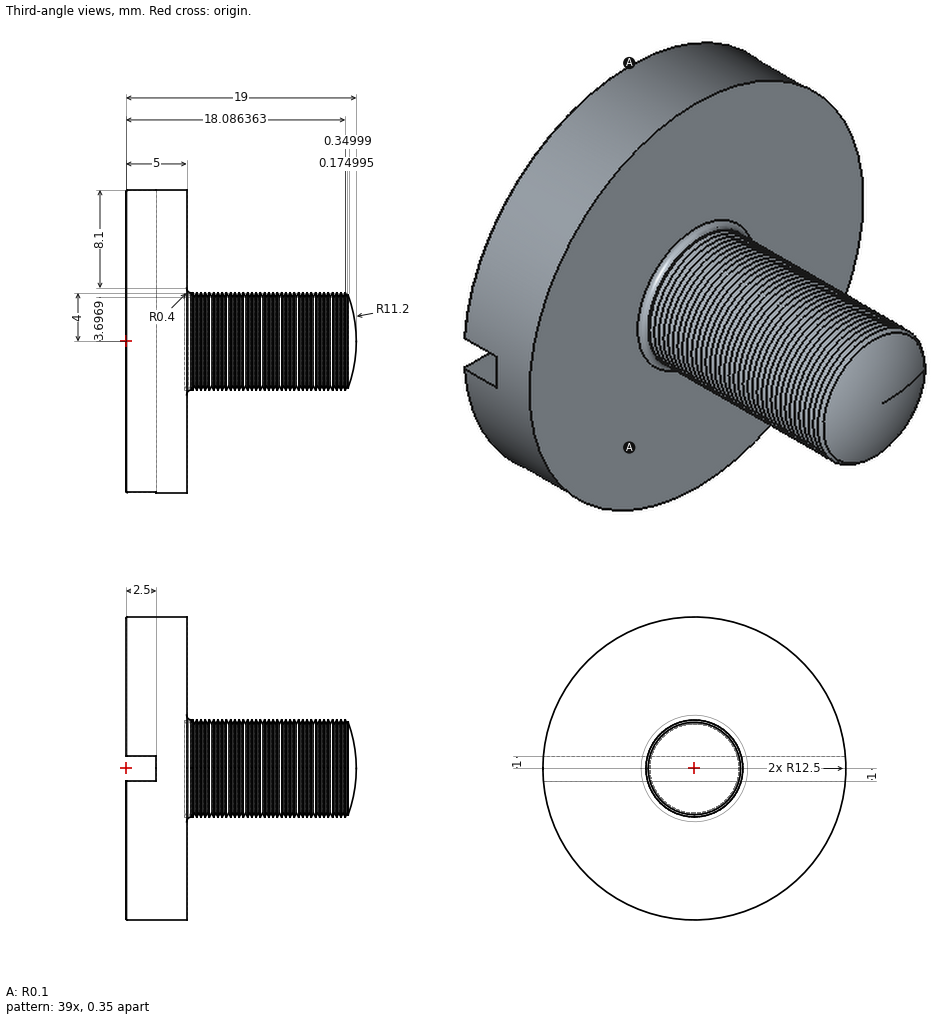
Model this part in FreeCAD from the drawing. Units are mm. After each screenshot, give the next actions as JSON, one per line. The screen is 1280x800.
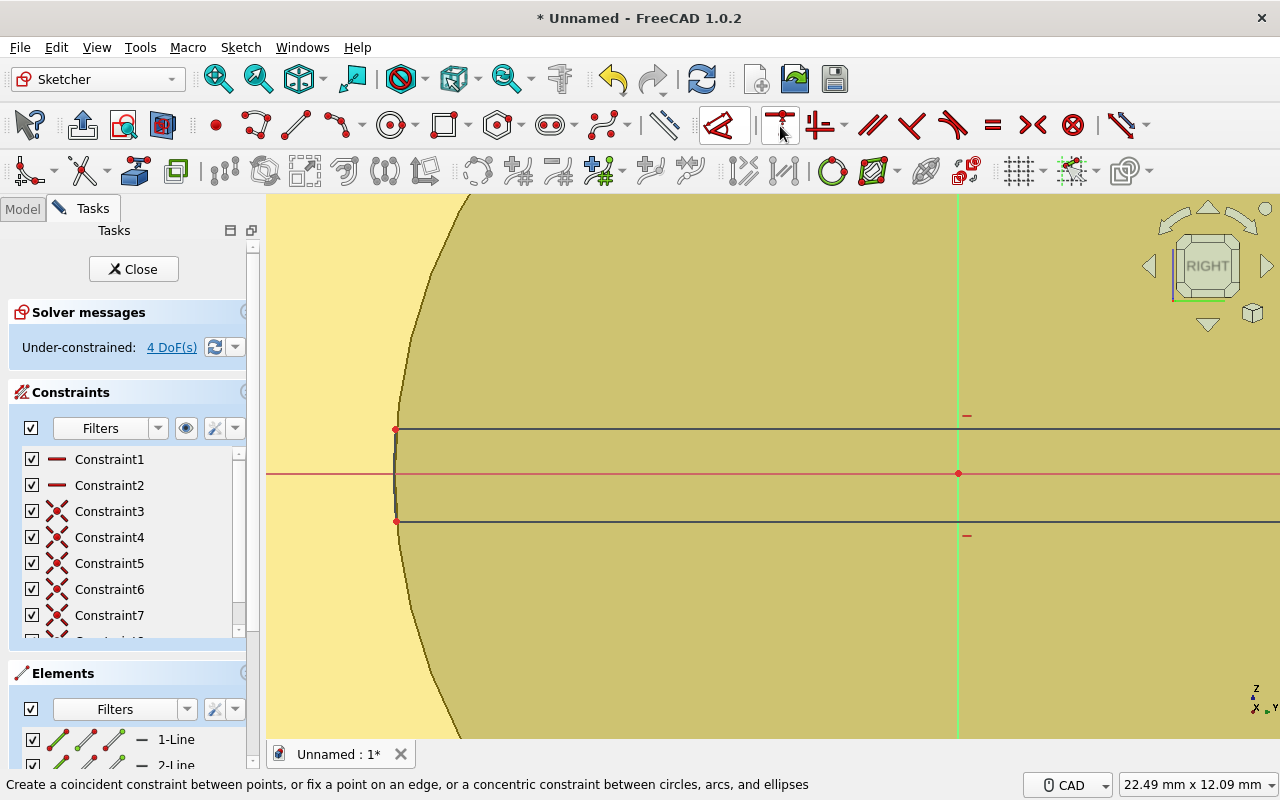
{"action": "scroll", "coordinate": [396, 458], "scroll_direction": "down", "scroll_amount": 3}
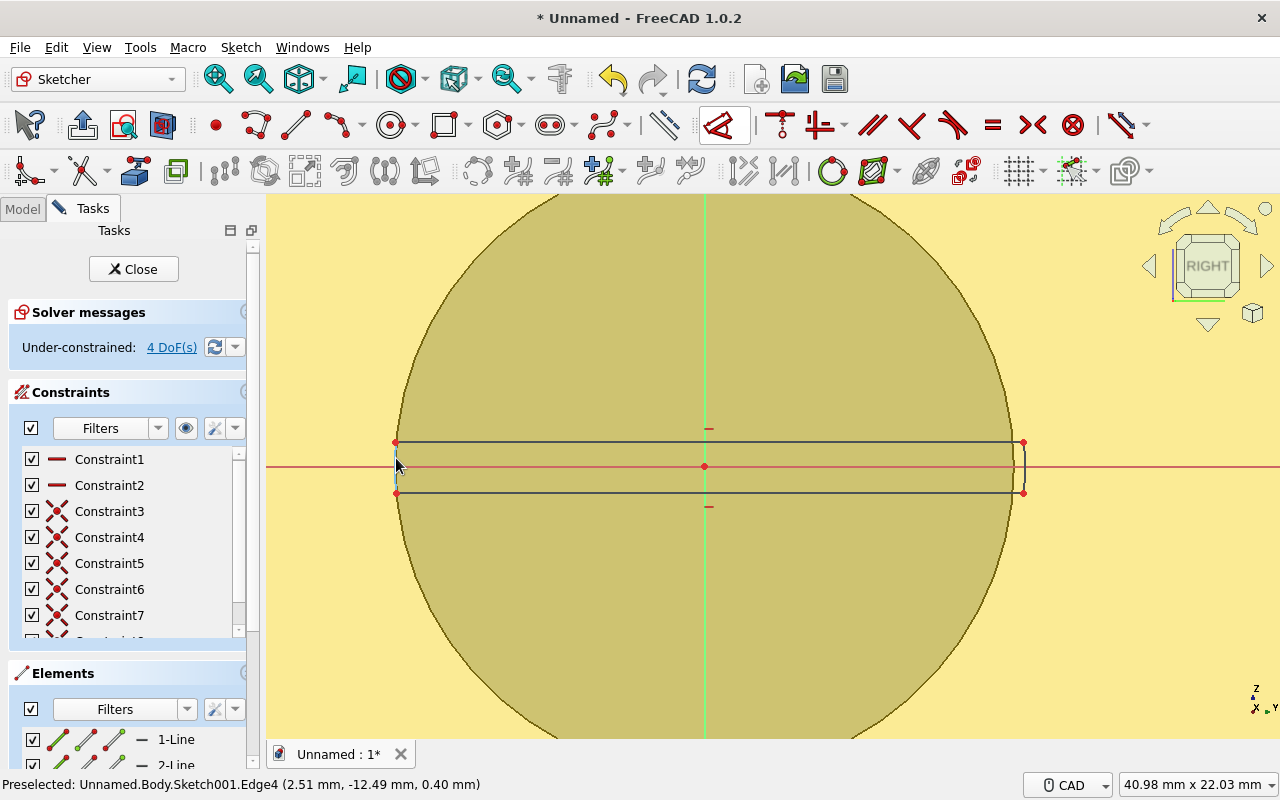
{"action": "scroll", "coordinate": [1025, 478], "scroll_direction": "up", "scroll_amount": 2}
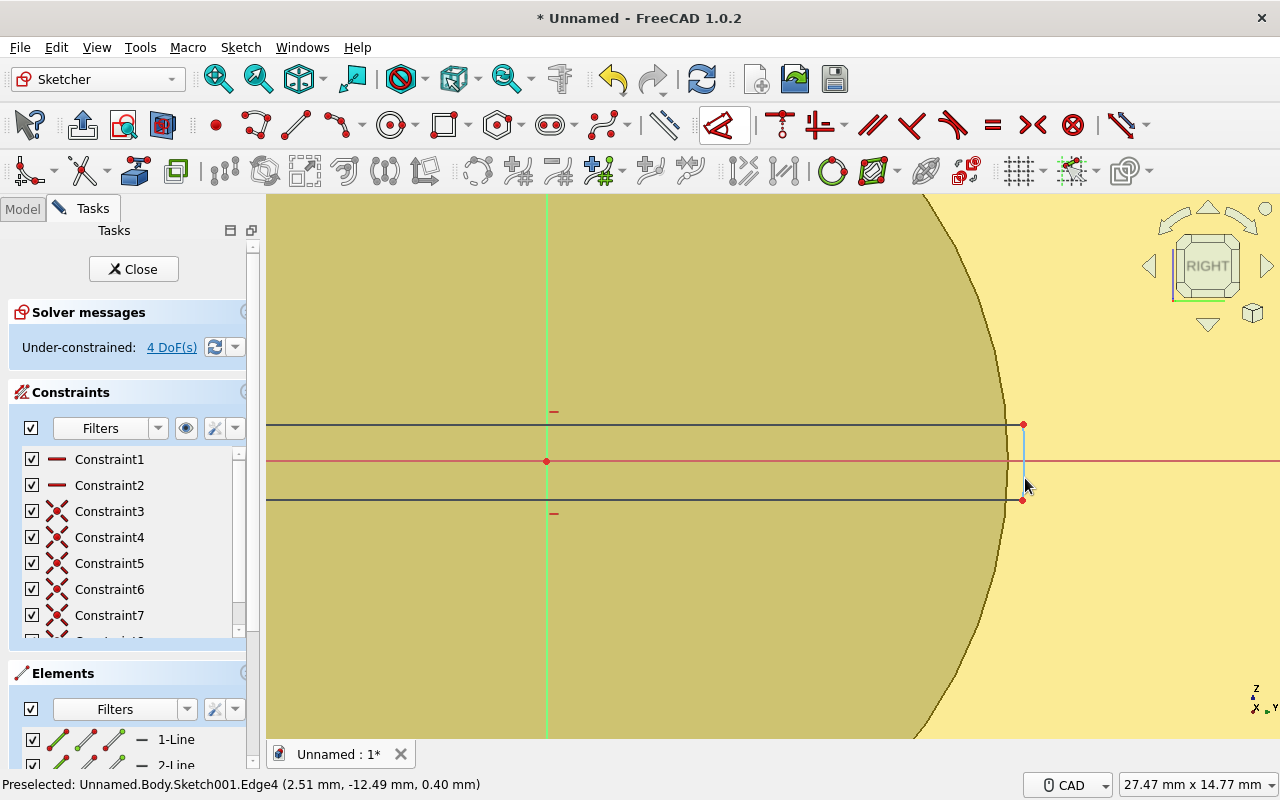
{"action": "left_click", "coordinate": [1024, 478]}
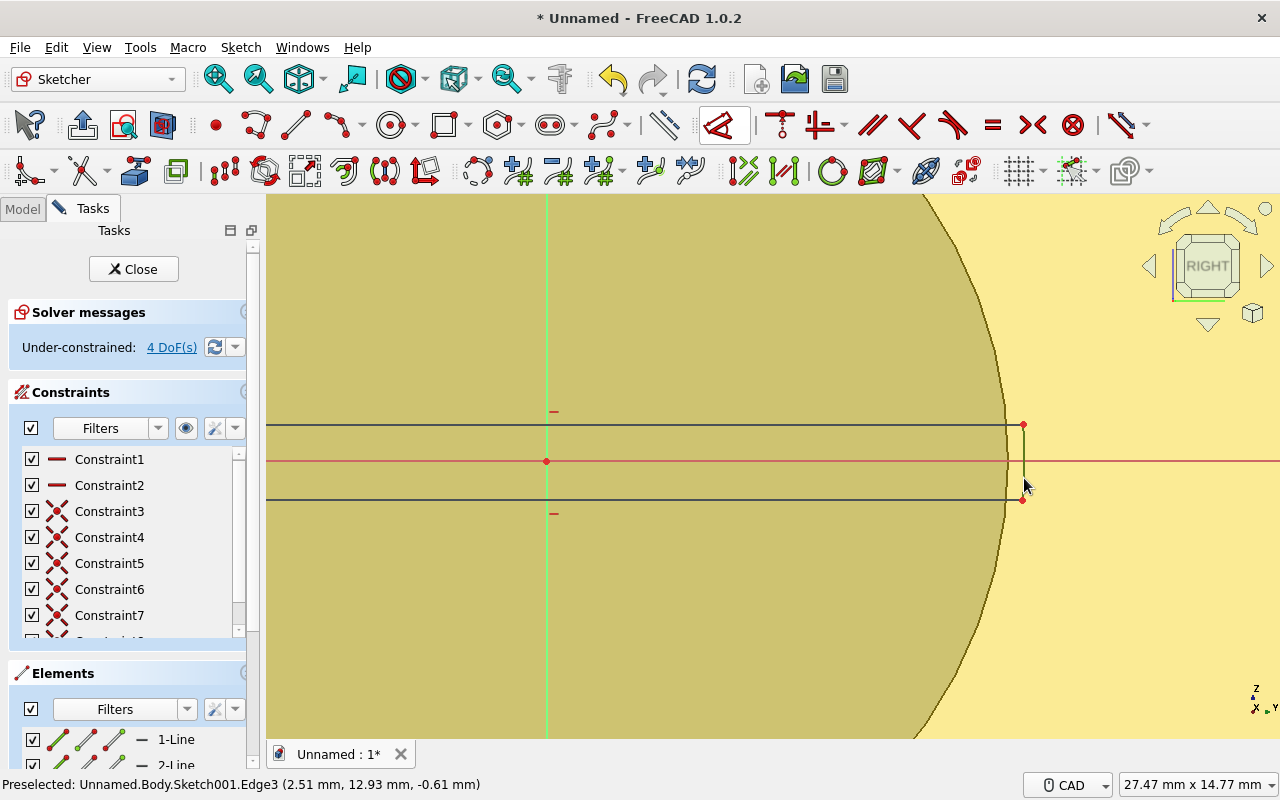
{"action": "scroll", "coordinate": [1025, 478], "scroll_direction": "down", "scroll_amount": 2}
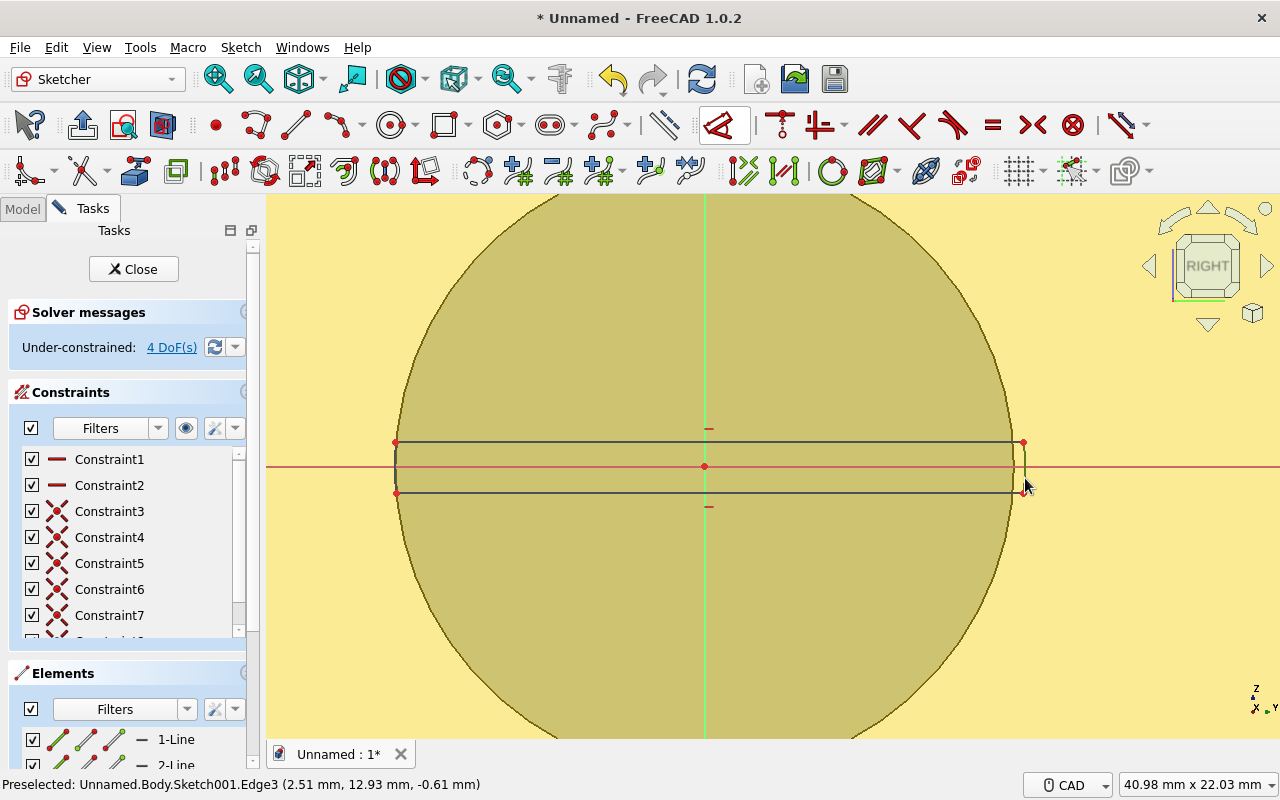
{"action": "scroll", "coordinate": [395, 458], "scroll_direction": "up", "scroll_amount": 3}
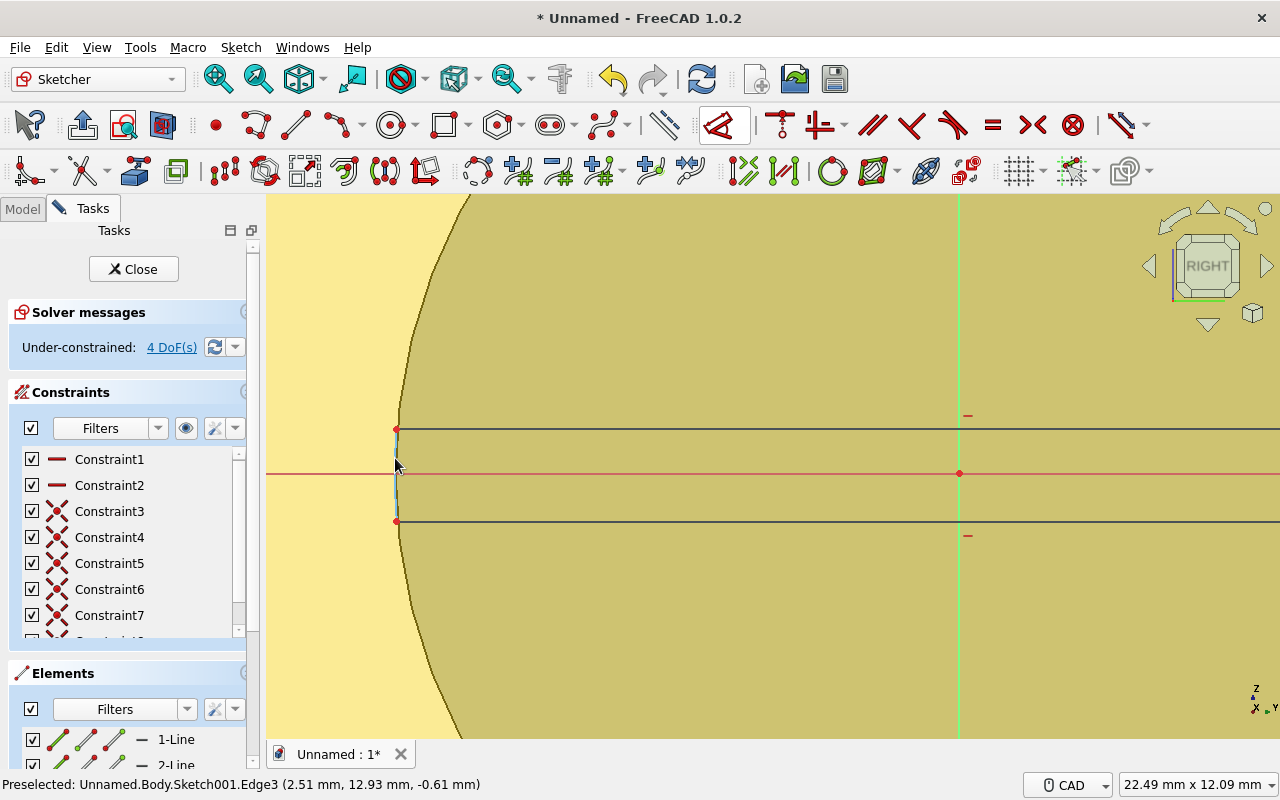
{"action": "left_click", "coordinate": [395, 457]}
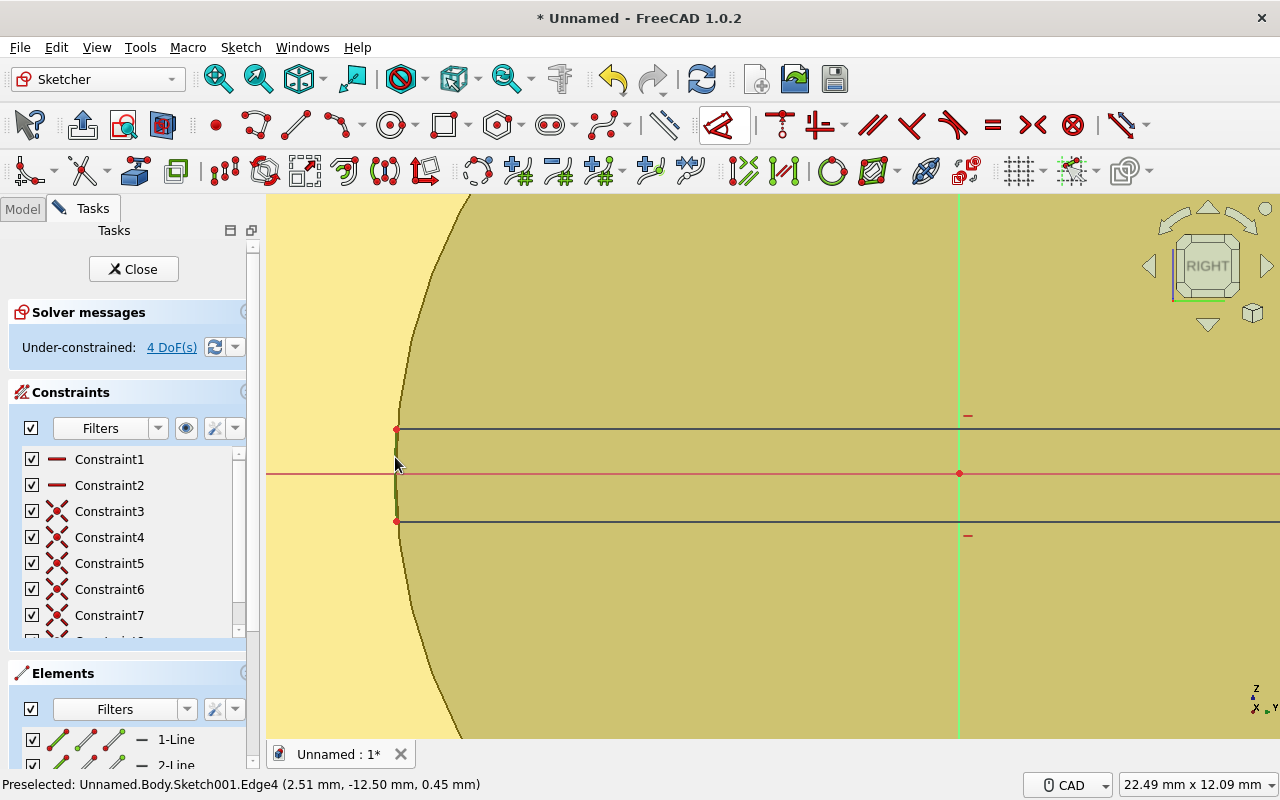
{"action": "left_click", "coordinate": [994, 126]}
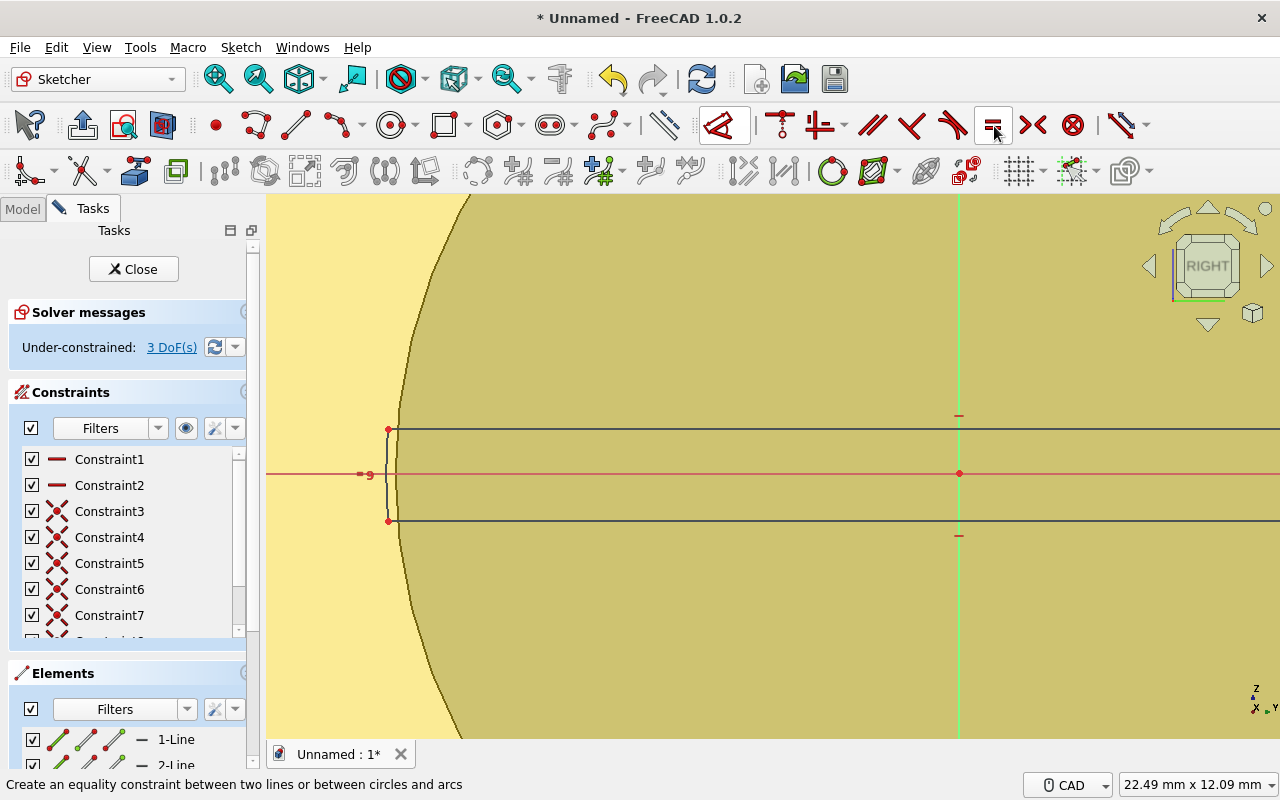
{"action": "scroll", "coordinate": [395, 458], "scroll_direction": "down", "scroll_amount": 3}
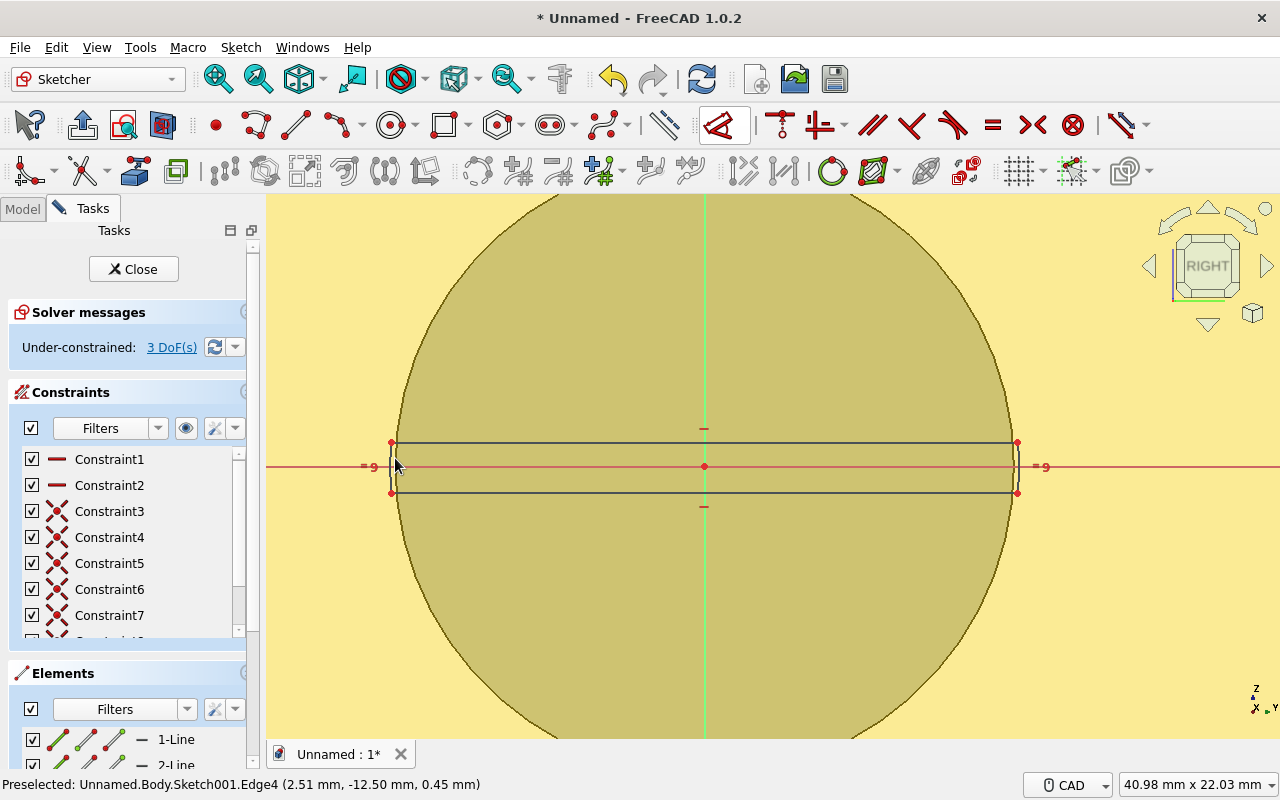
{"action": "scroll", "coordinate": [1019, 478], "scroll_direction": "up", "scroll_amount": 2}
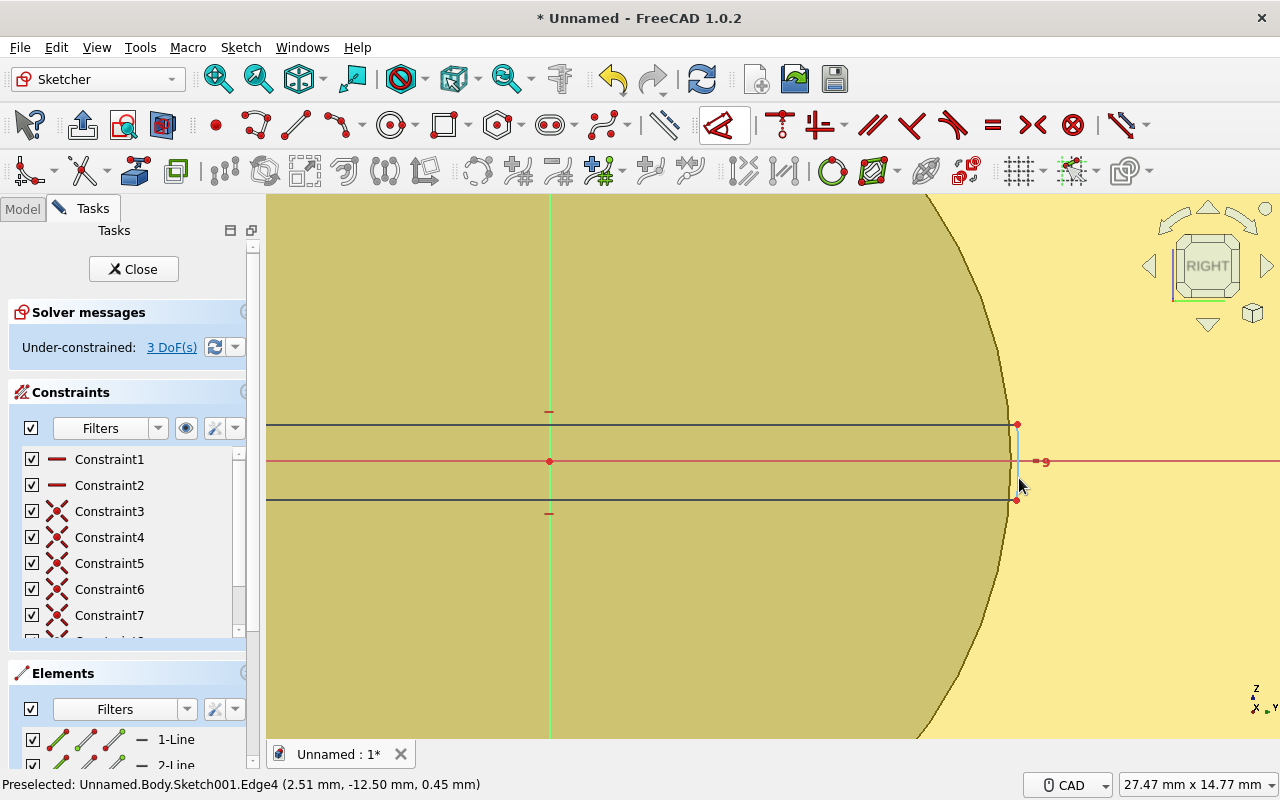
{"action": "left_click", "coordinate": [1018, 478]}